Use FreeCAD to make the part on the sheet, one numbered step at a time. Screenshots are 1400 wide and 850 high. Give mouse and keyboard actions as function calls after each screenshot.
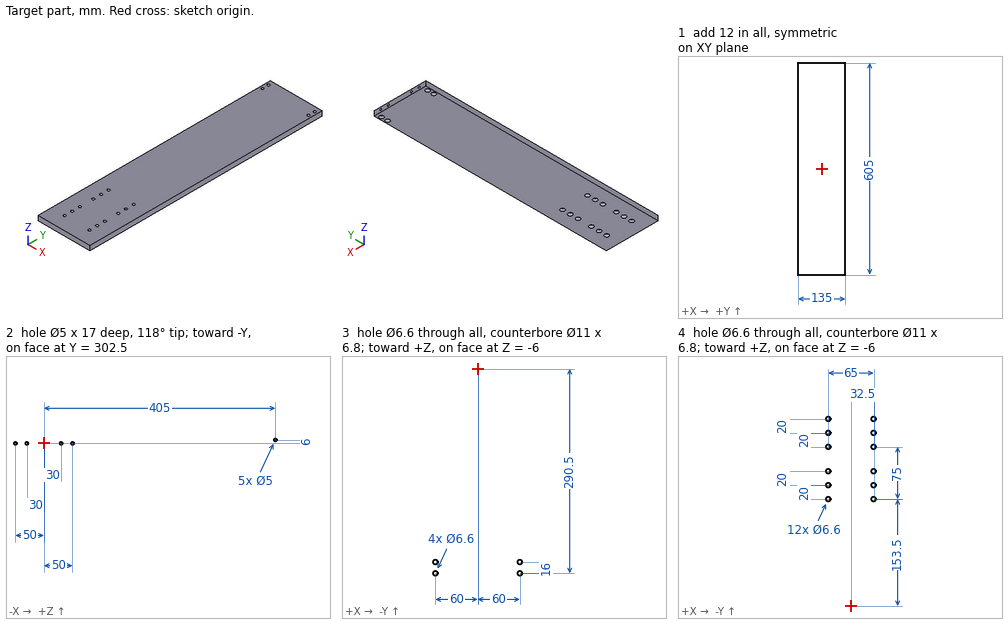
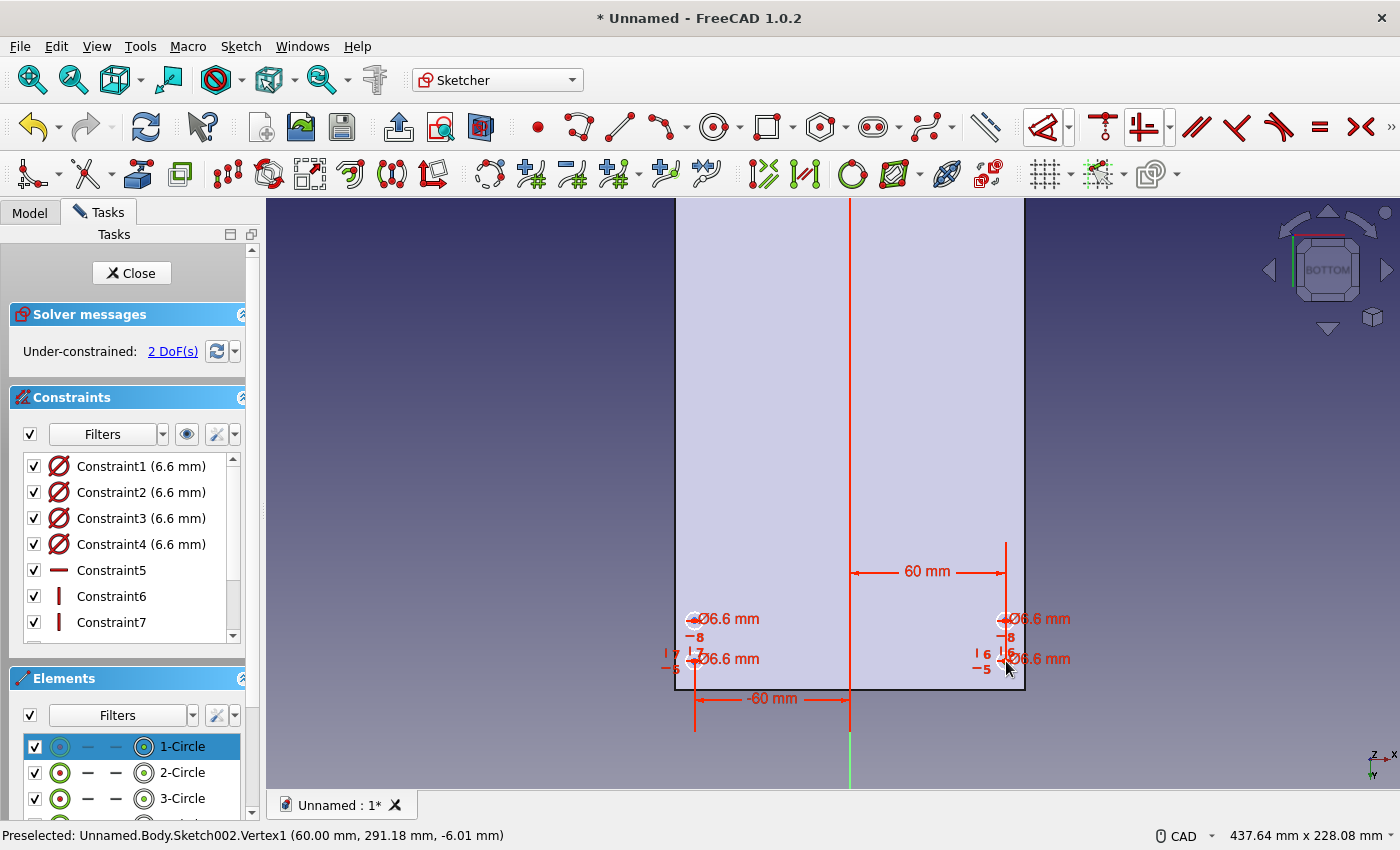
click(1006, 621)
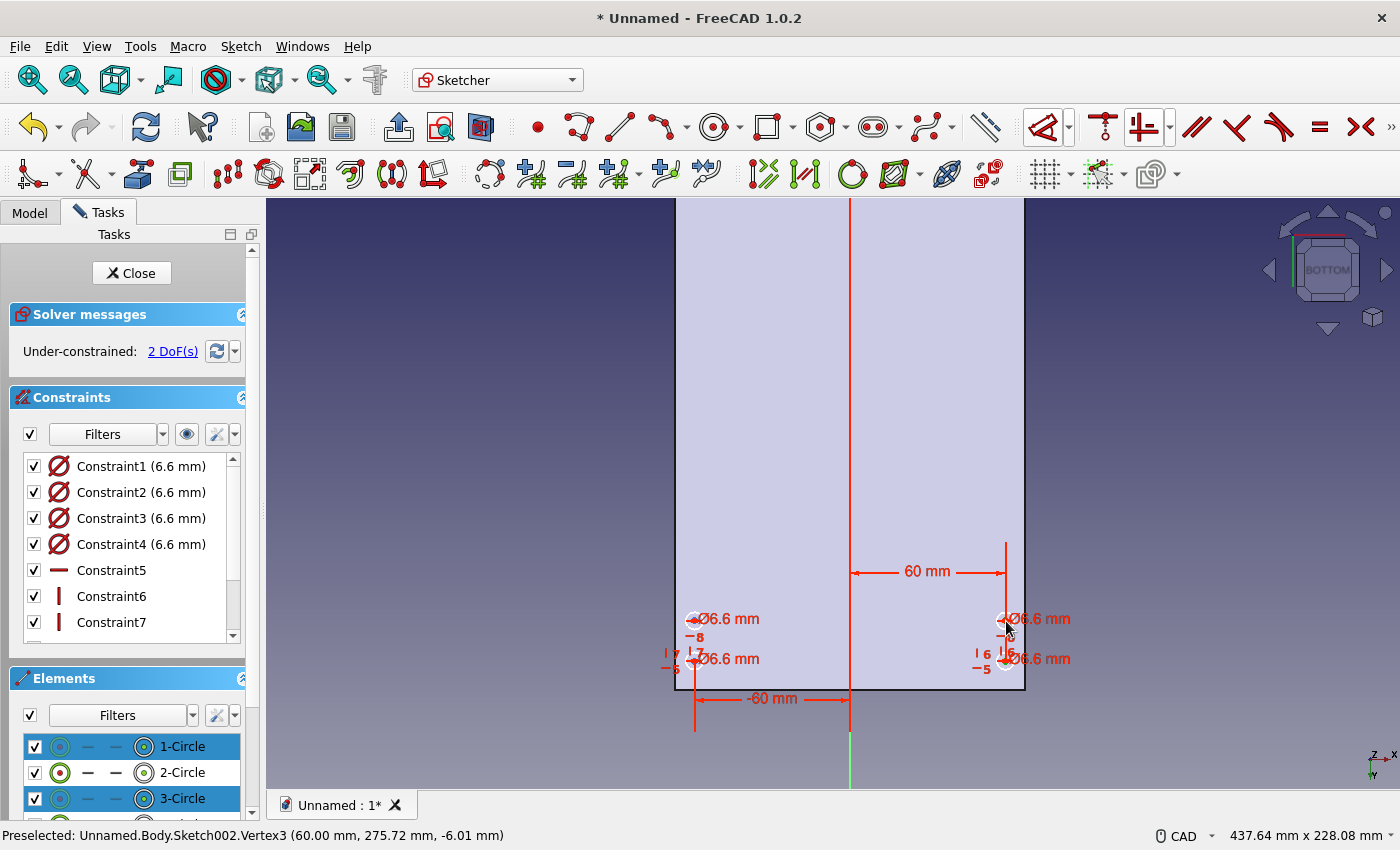
key(i)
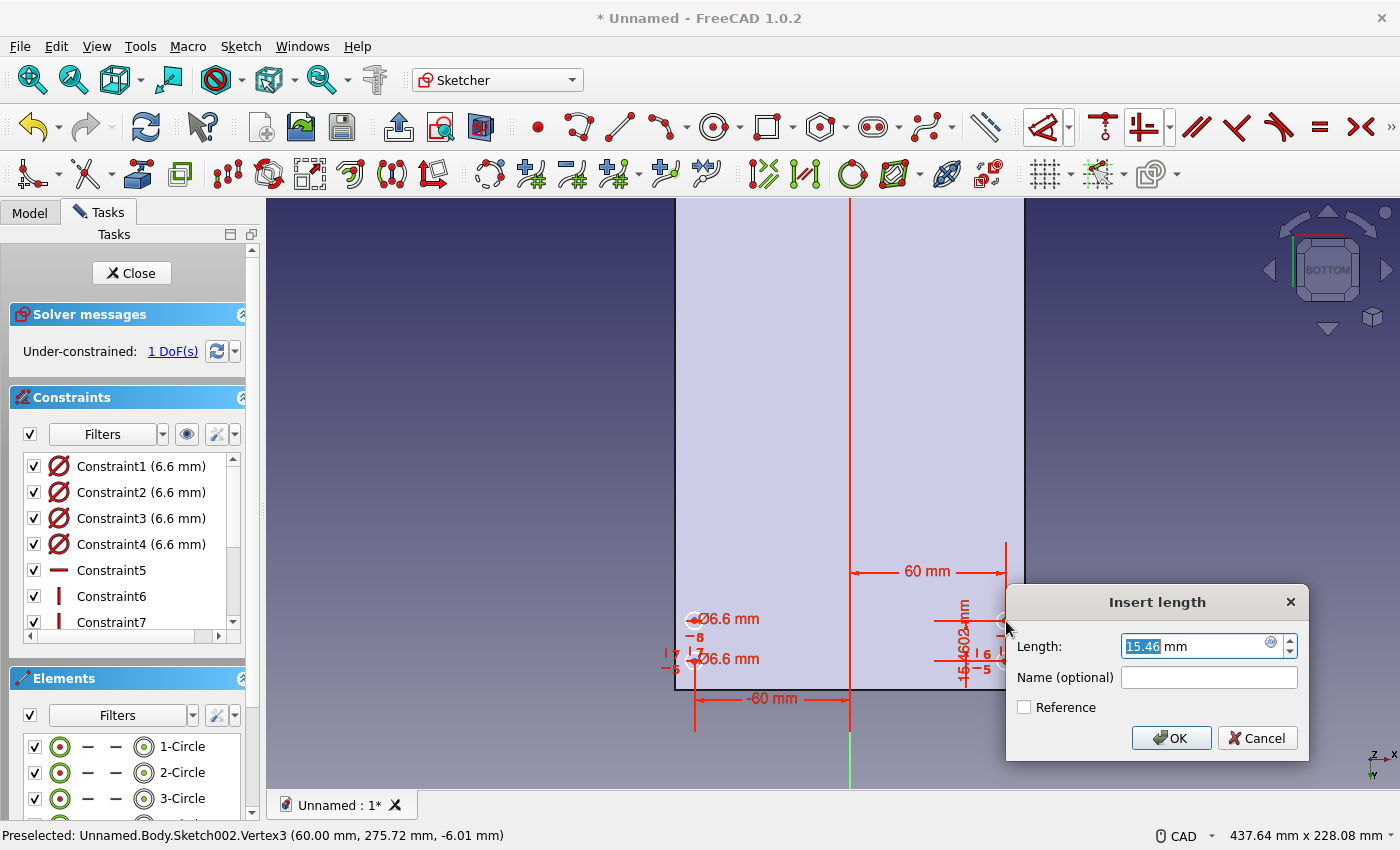
text(16)
key(Return)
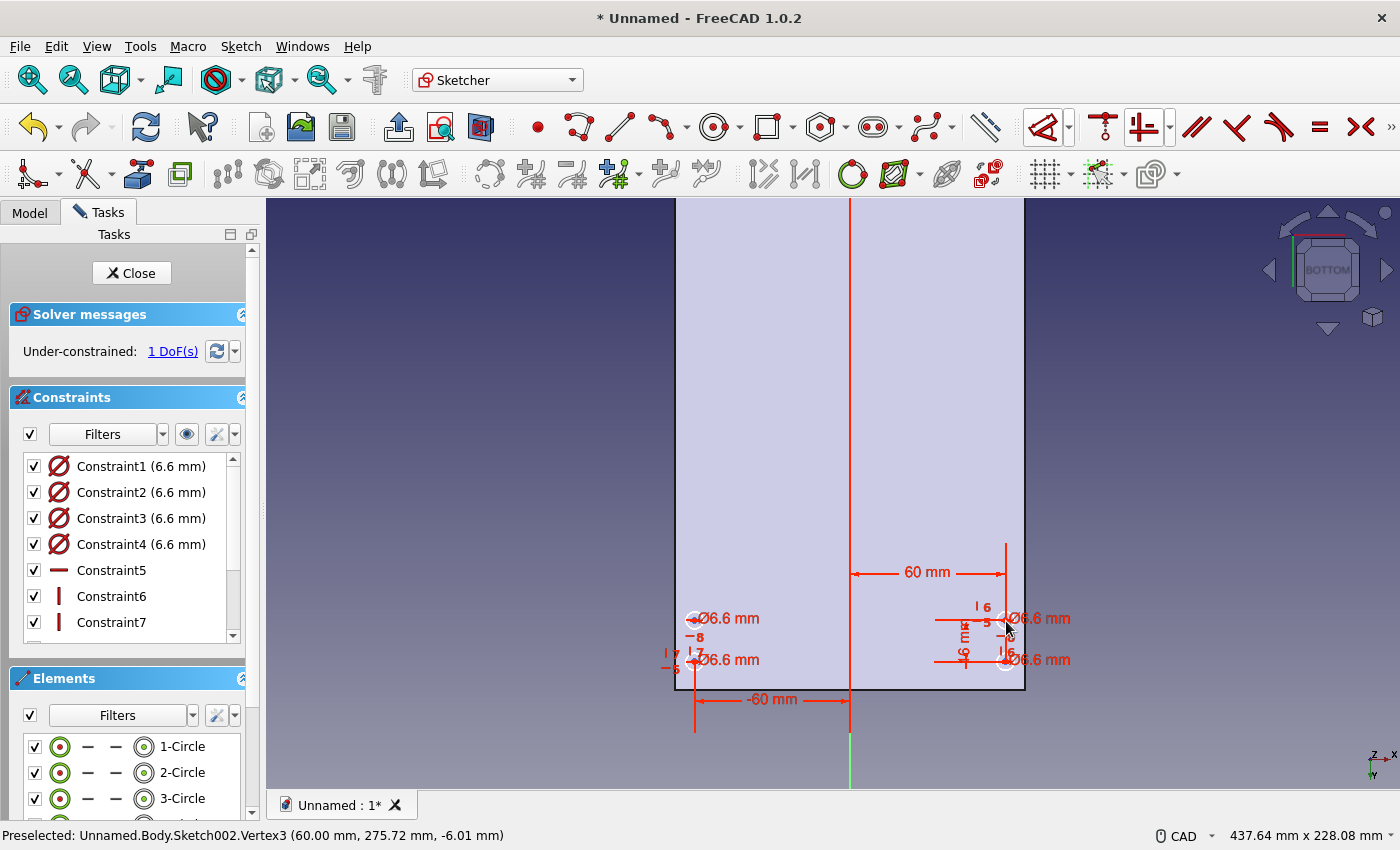
click(1006, 662)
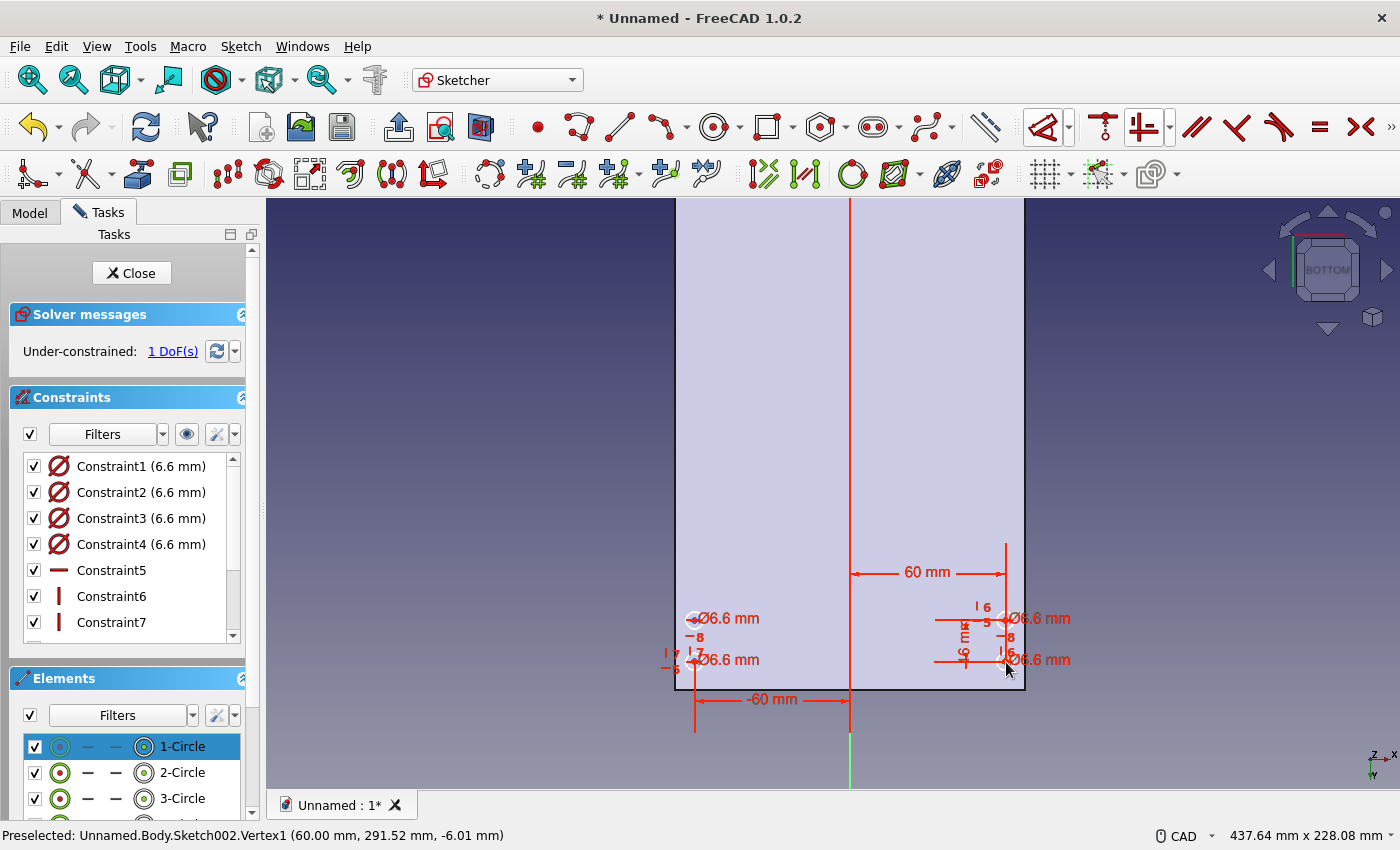
click(1068, 128)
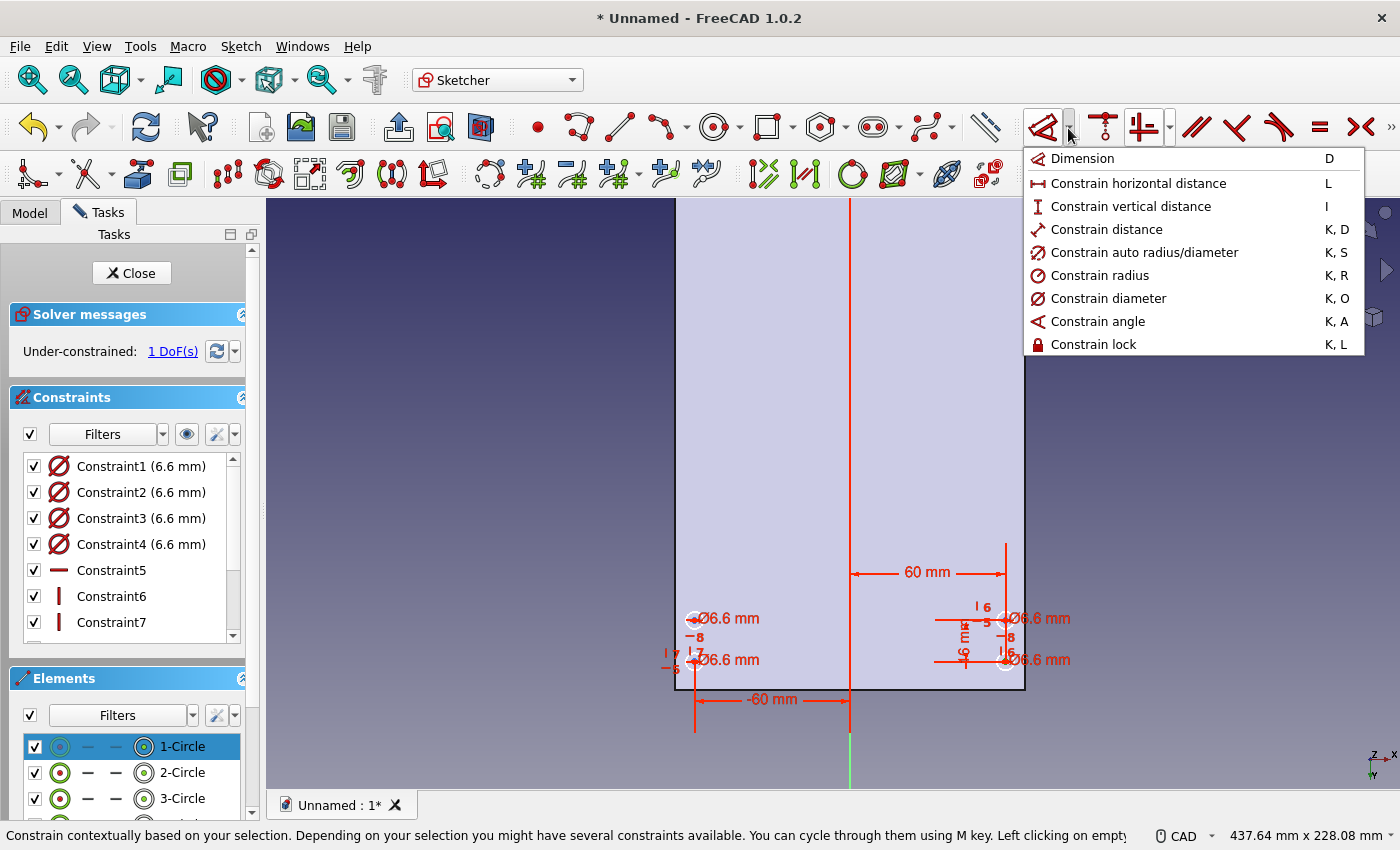
click(1194, 206)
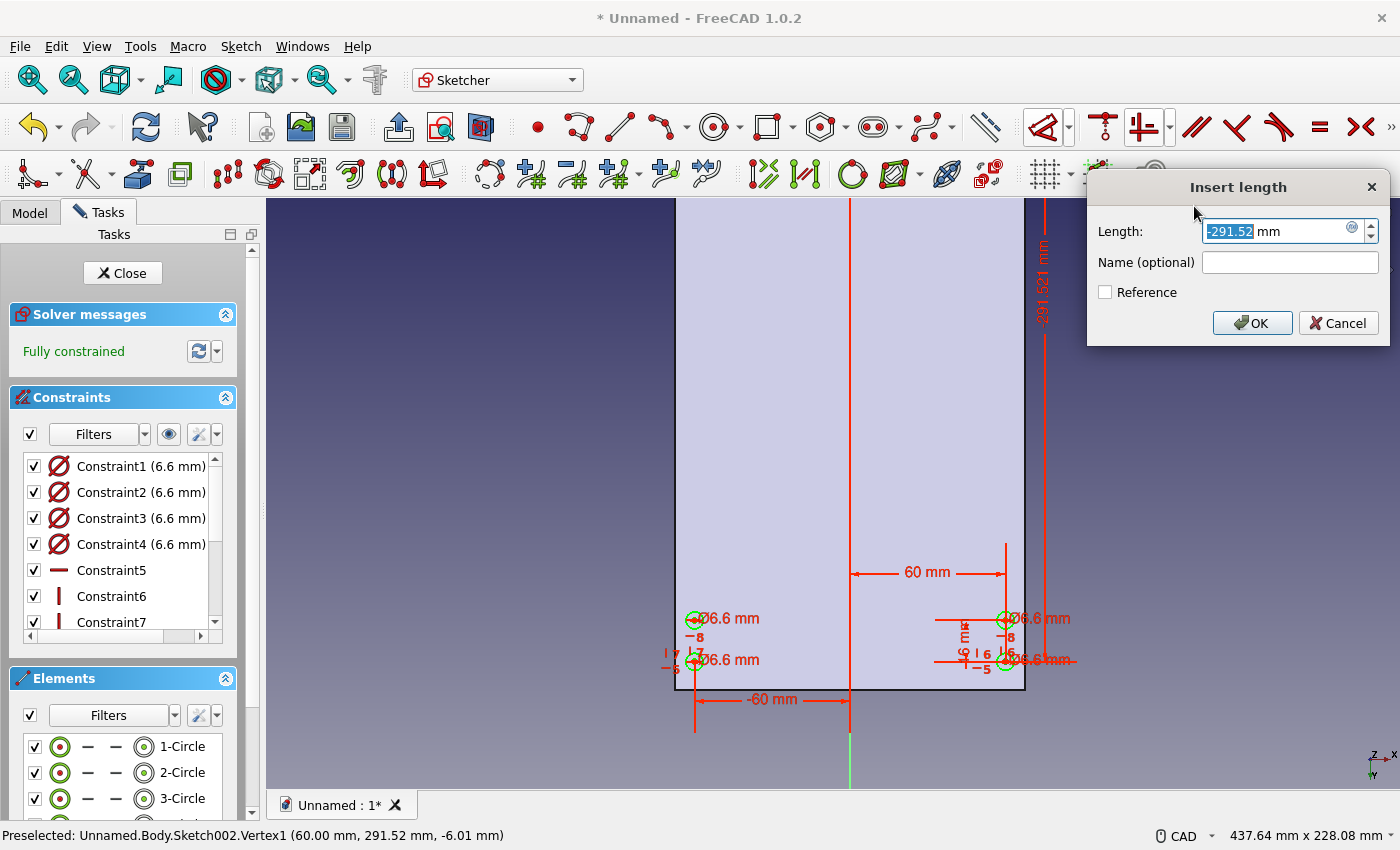
text(-290.5)
key(Return)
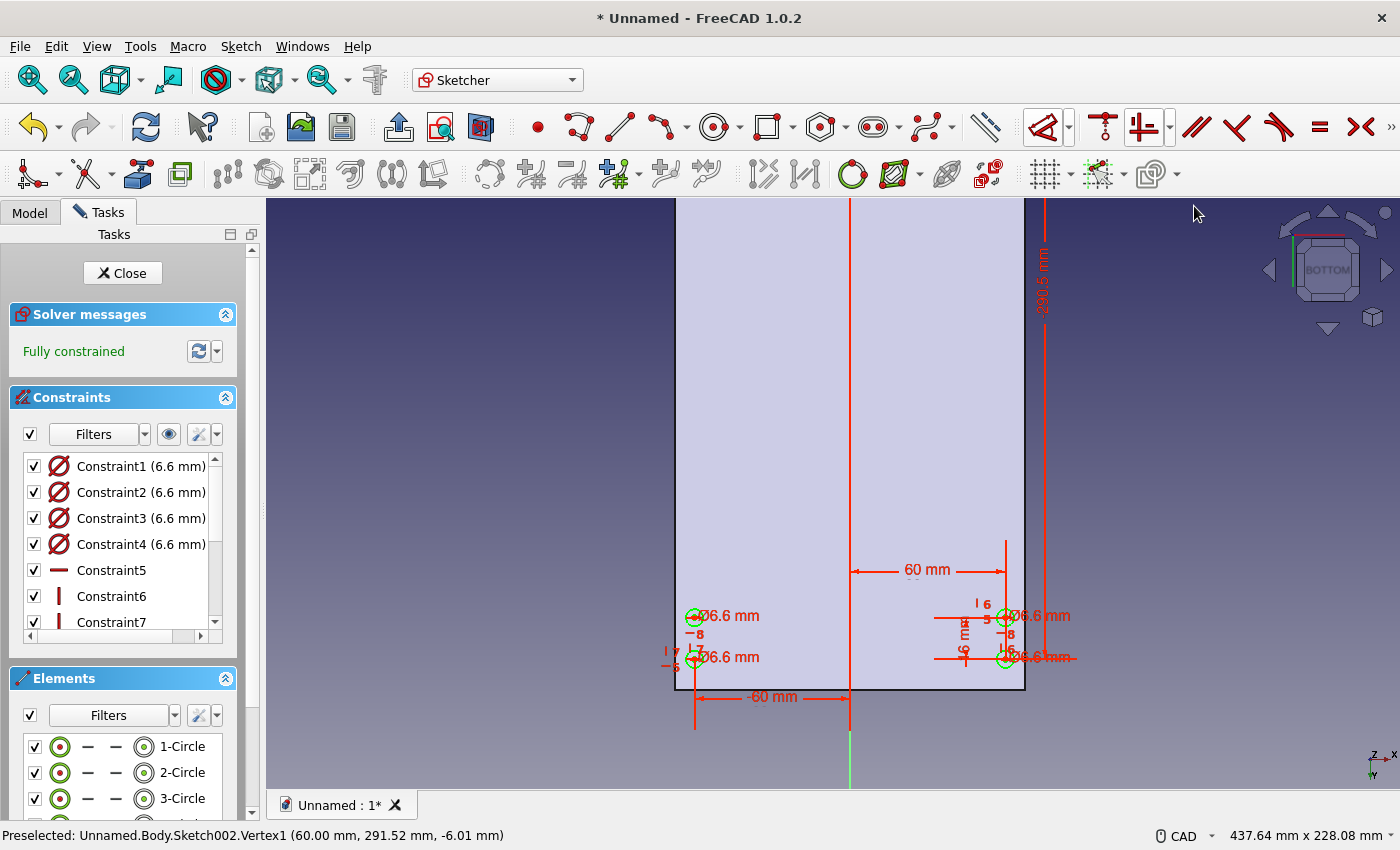
click(123, 273)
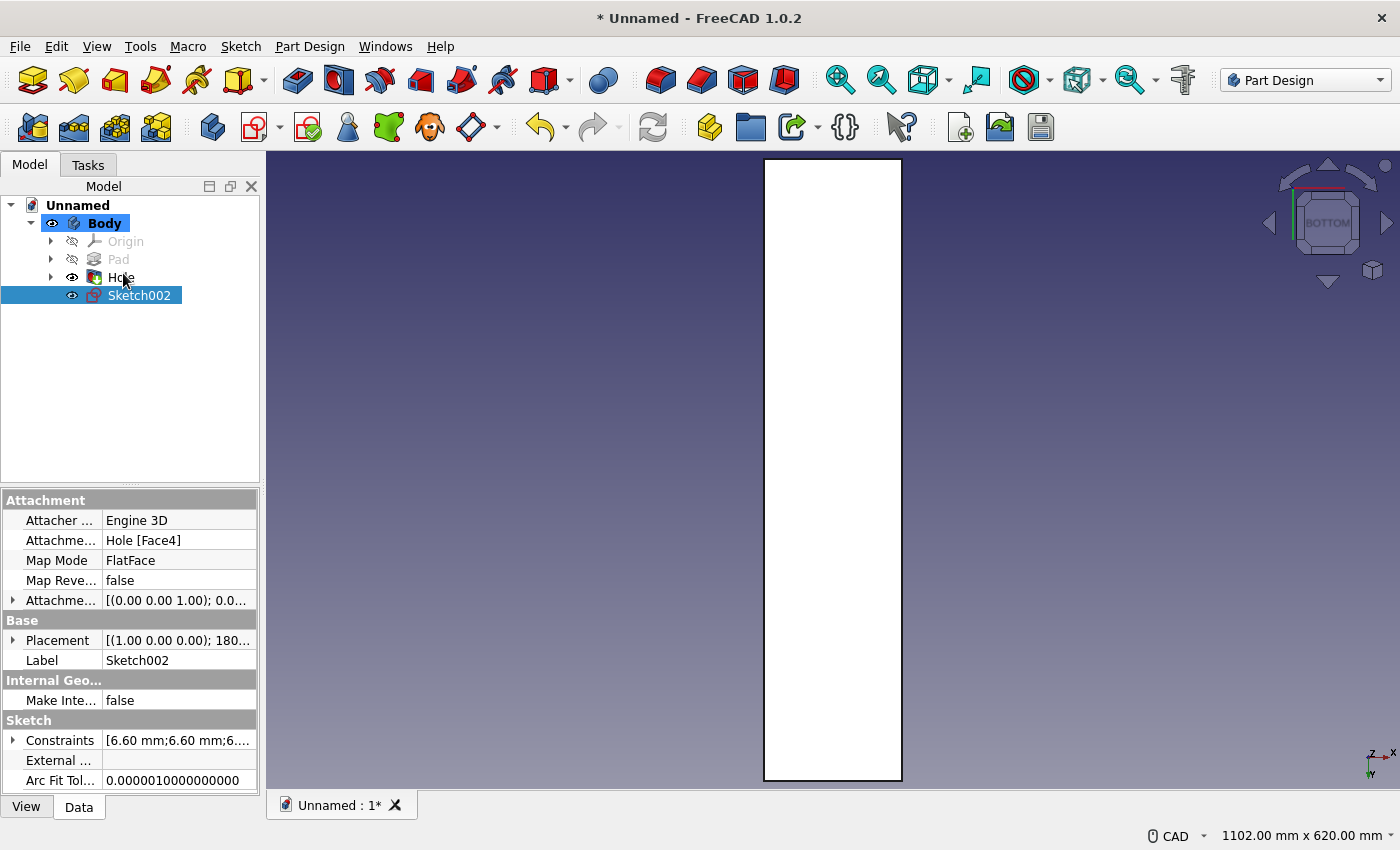
click(339, 80)